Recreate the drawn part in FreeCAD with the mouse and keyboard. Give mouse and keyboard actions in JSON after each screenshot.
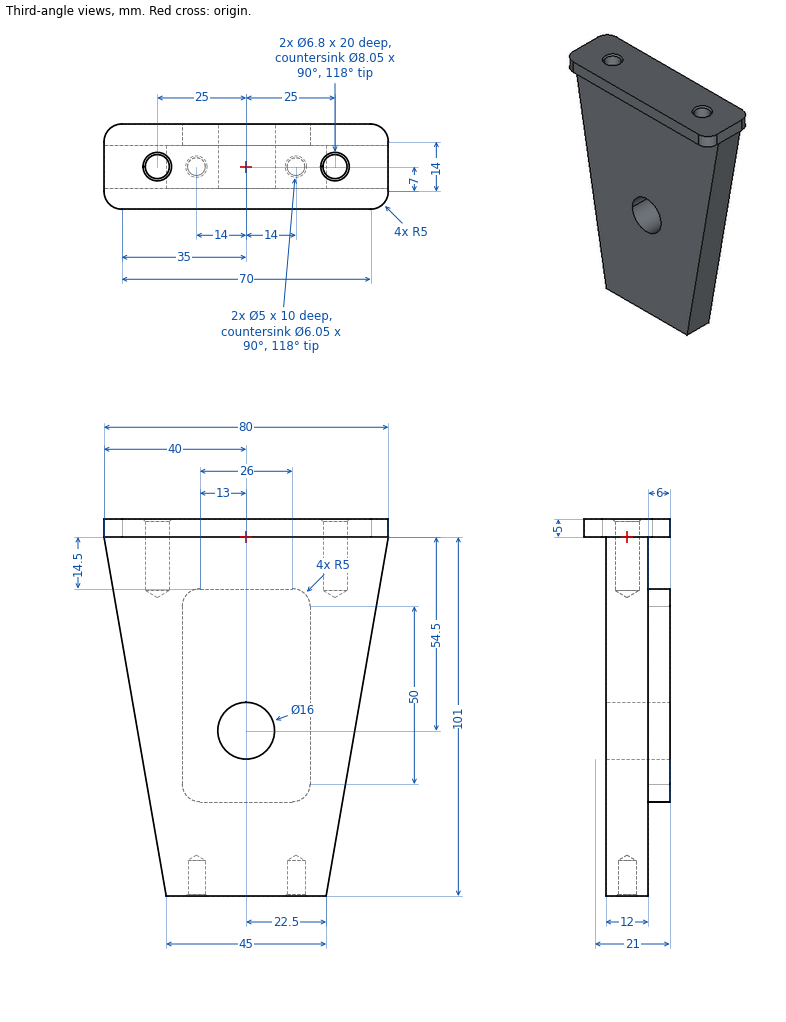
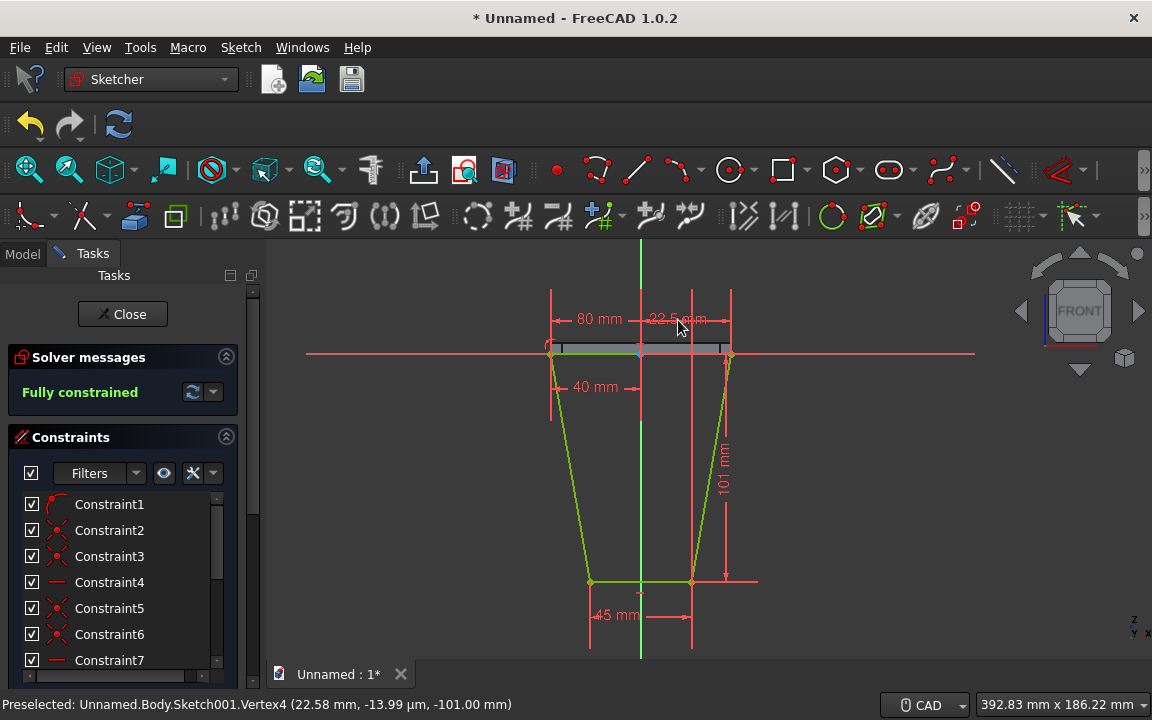
{"action": "left_click", "coordinate": [123, 314]}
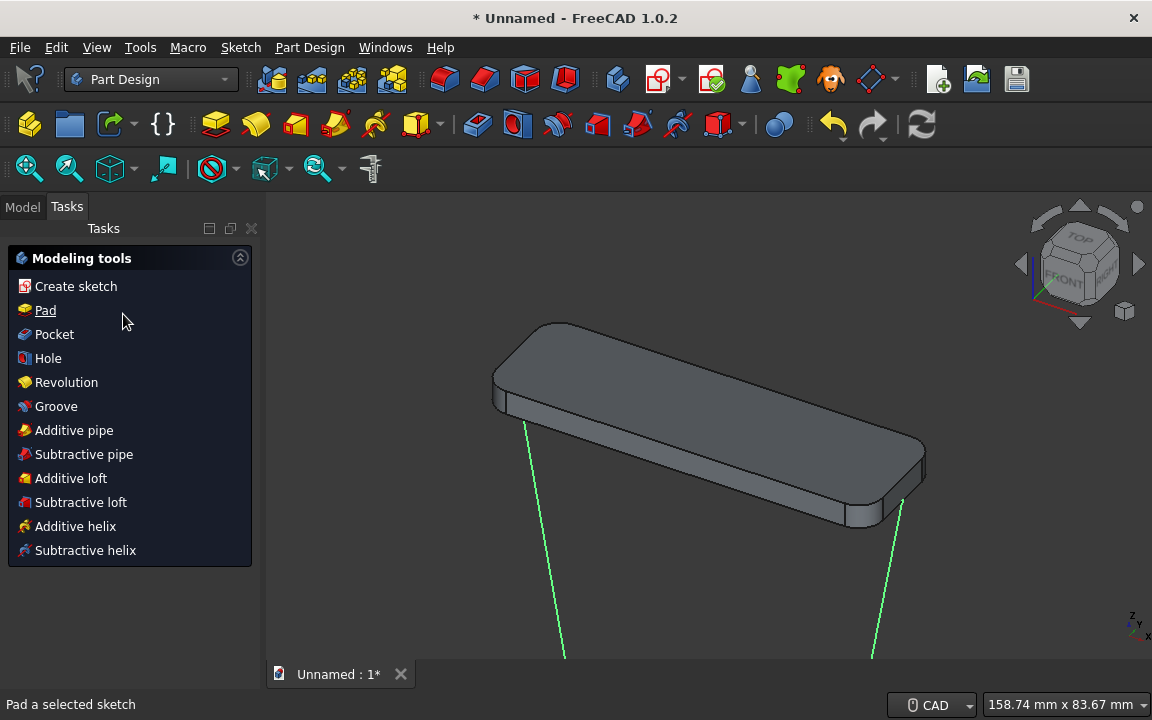
{"action": "left_click", "coordinate": [216, 124]}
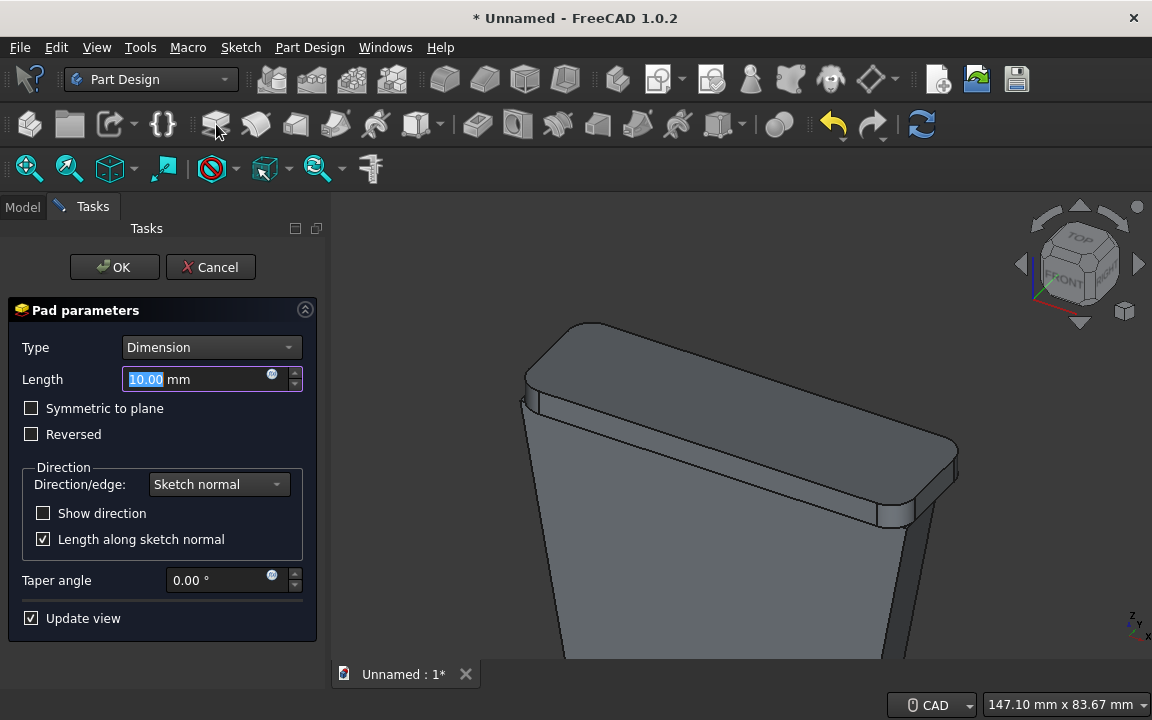
{"action": "type", "text": "12"}
{"action": "key", "text": "Tab"}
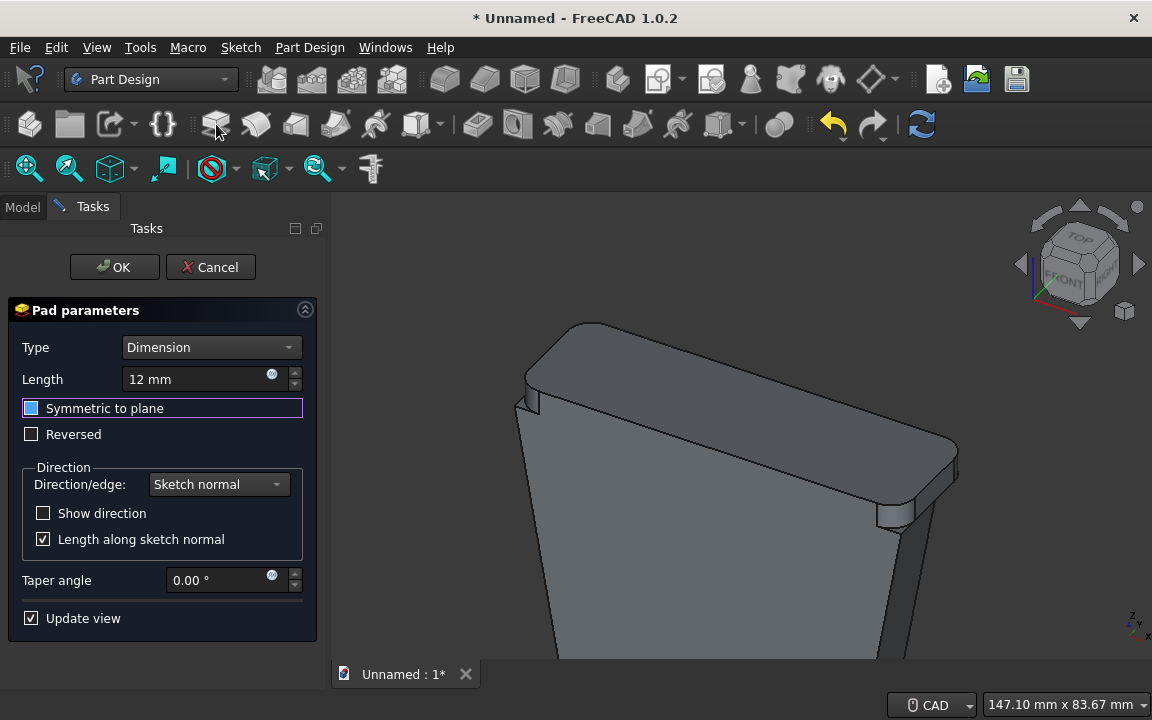
{"action": "left_click", "coordinate": [30, 408]}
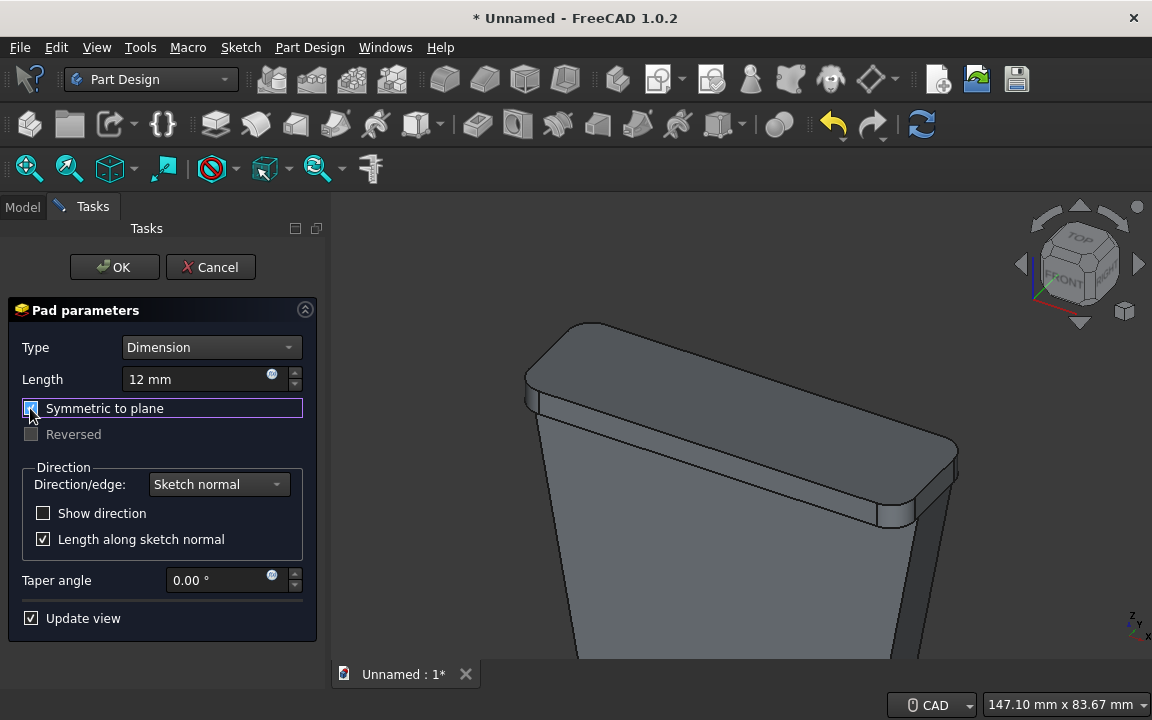
{"action": "left_click", "coordinate": [115, 267]}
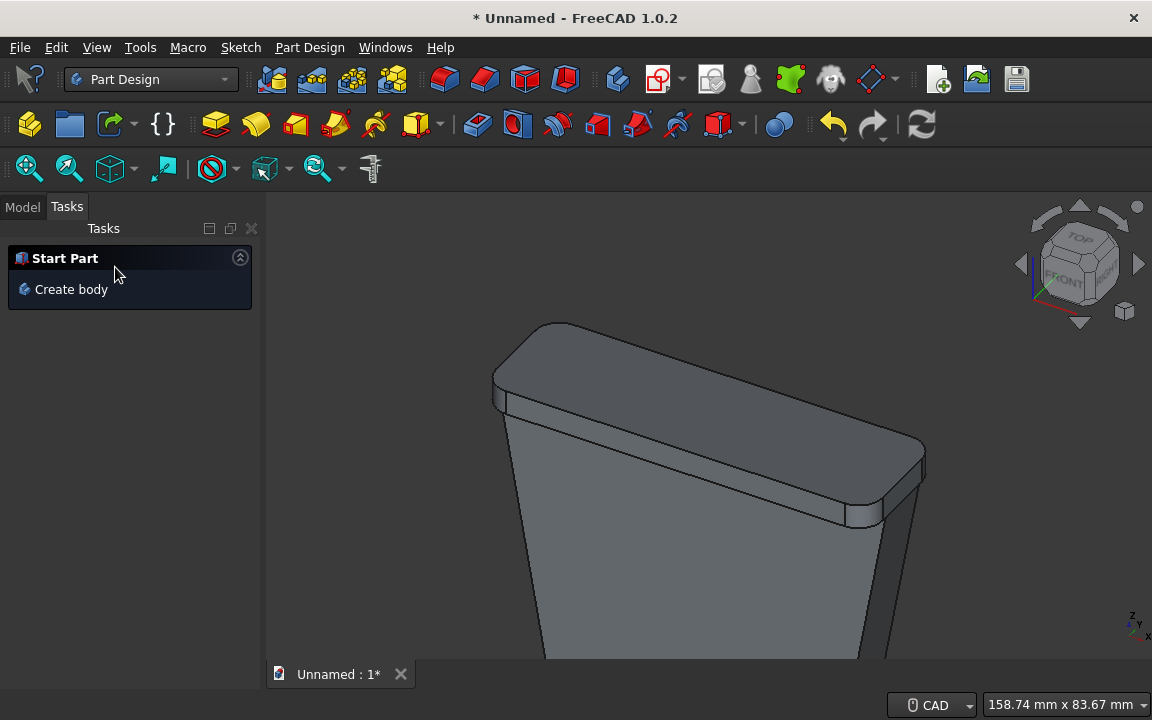
{"action": "left_click", "coordinate": [30, 170]}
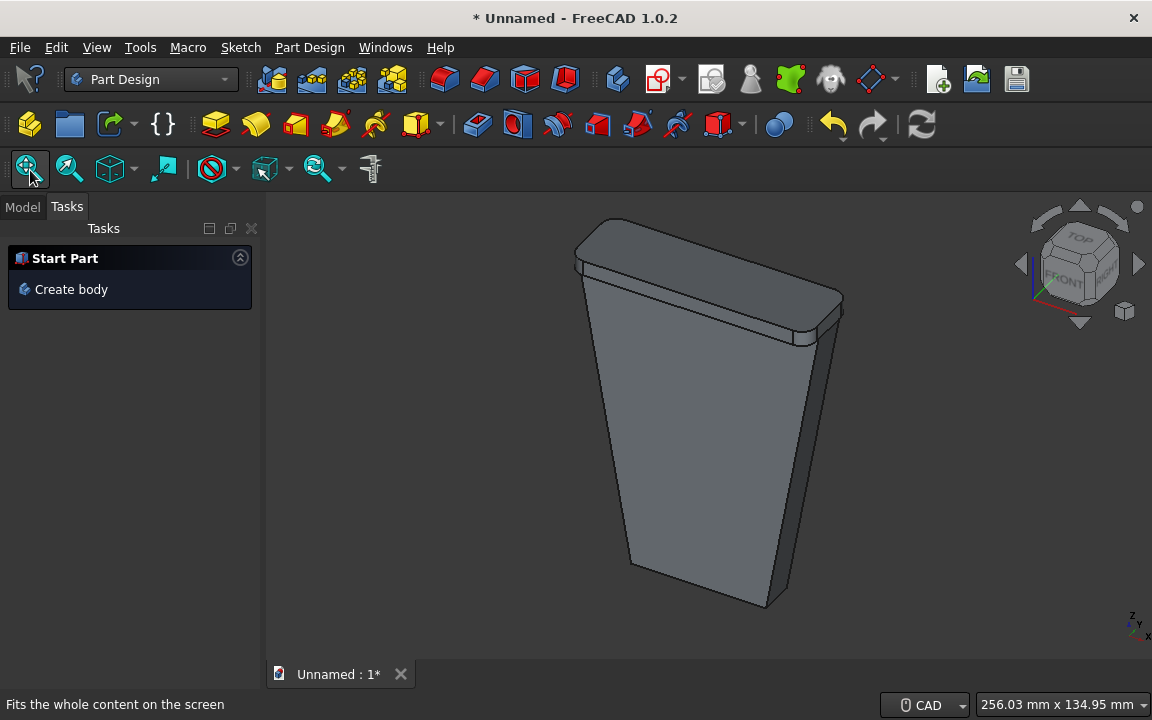
{"action": "key", "text": "4"}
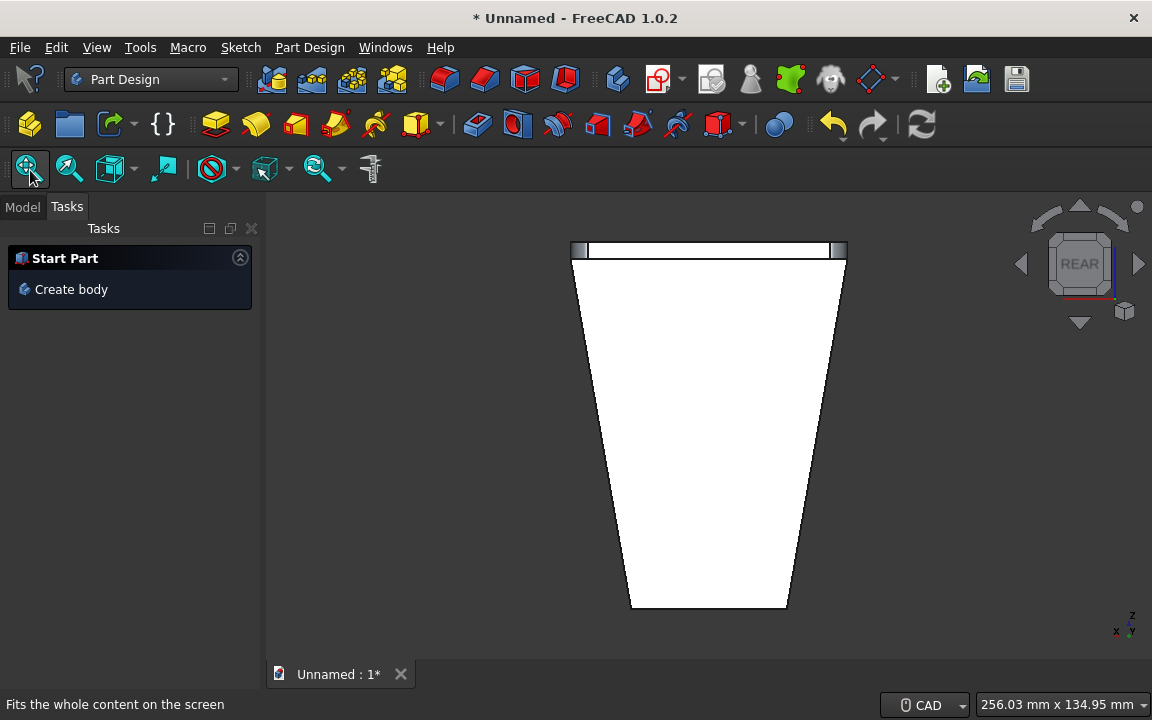
{"action": "left_click", "coordinate": [709, 383]}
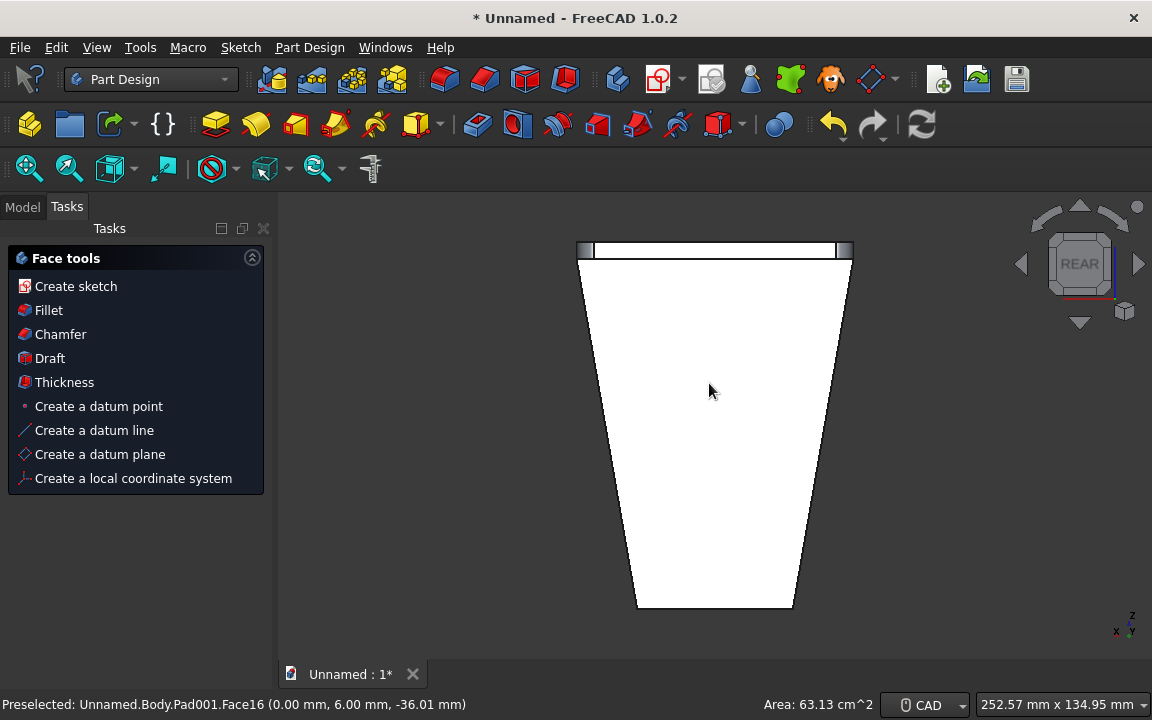
{"action": "left_click", "coordinate": [658, 80]}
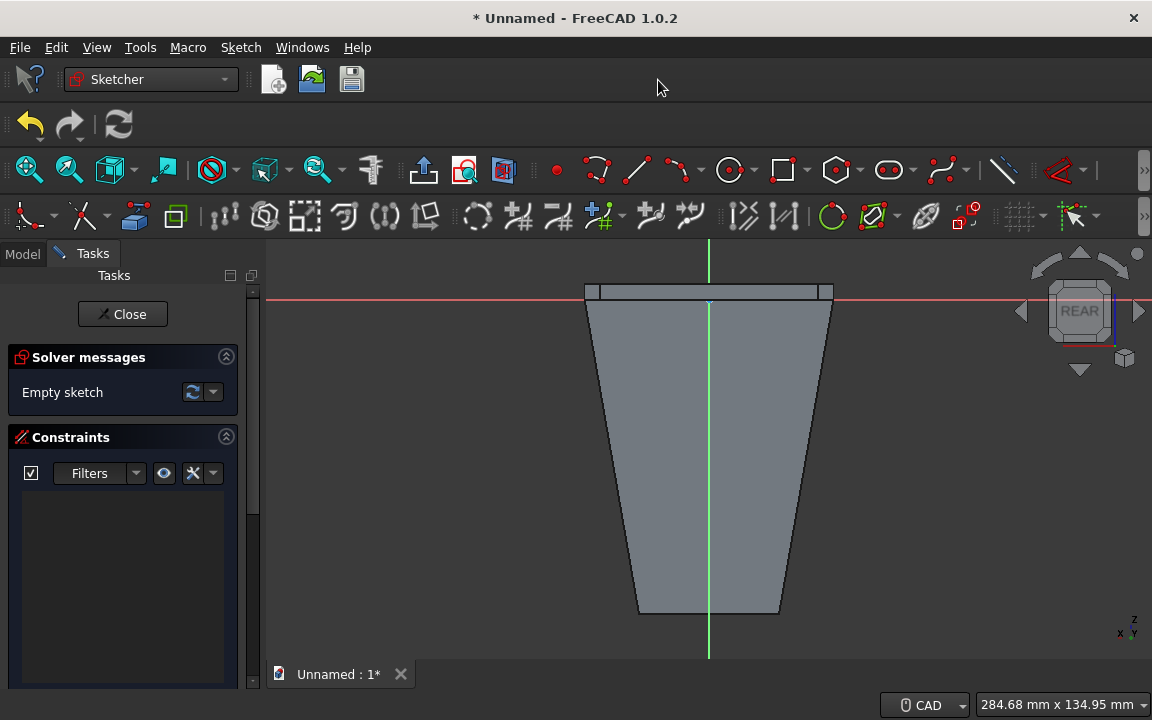
{"action": "left_click", "coordinate": [504, 170]}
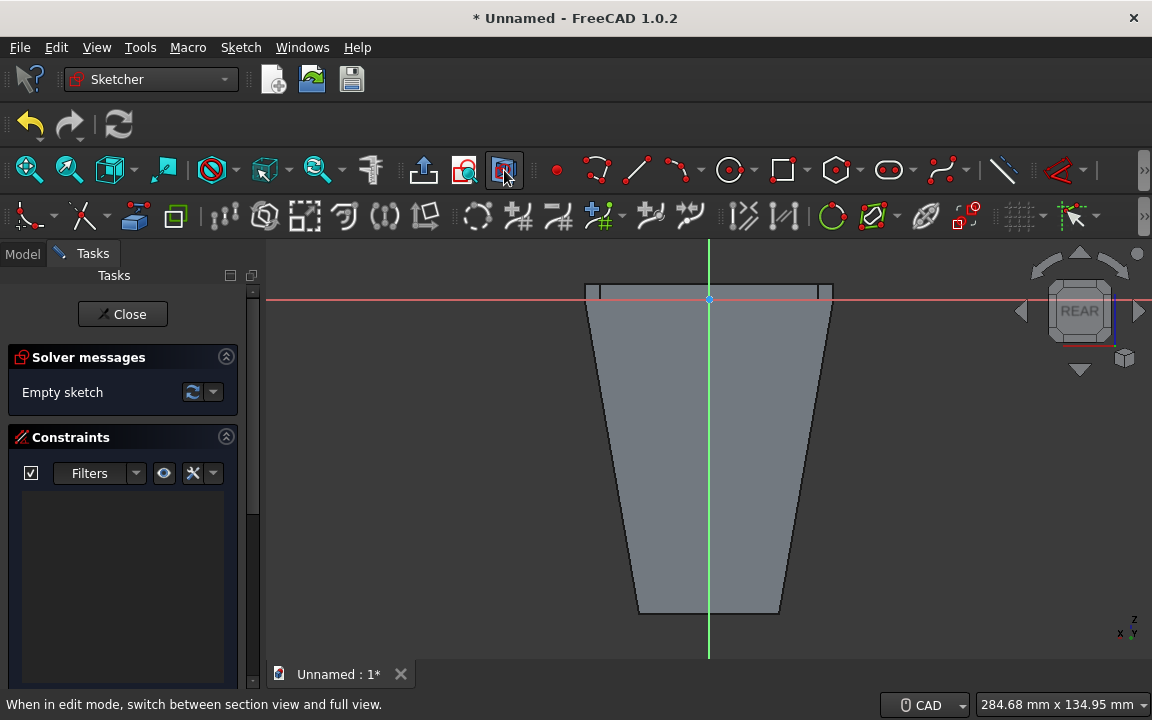
{"action": "left_click", "coordinate": [638, 170]}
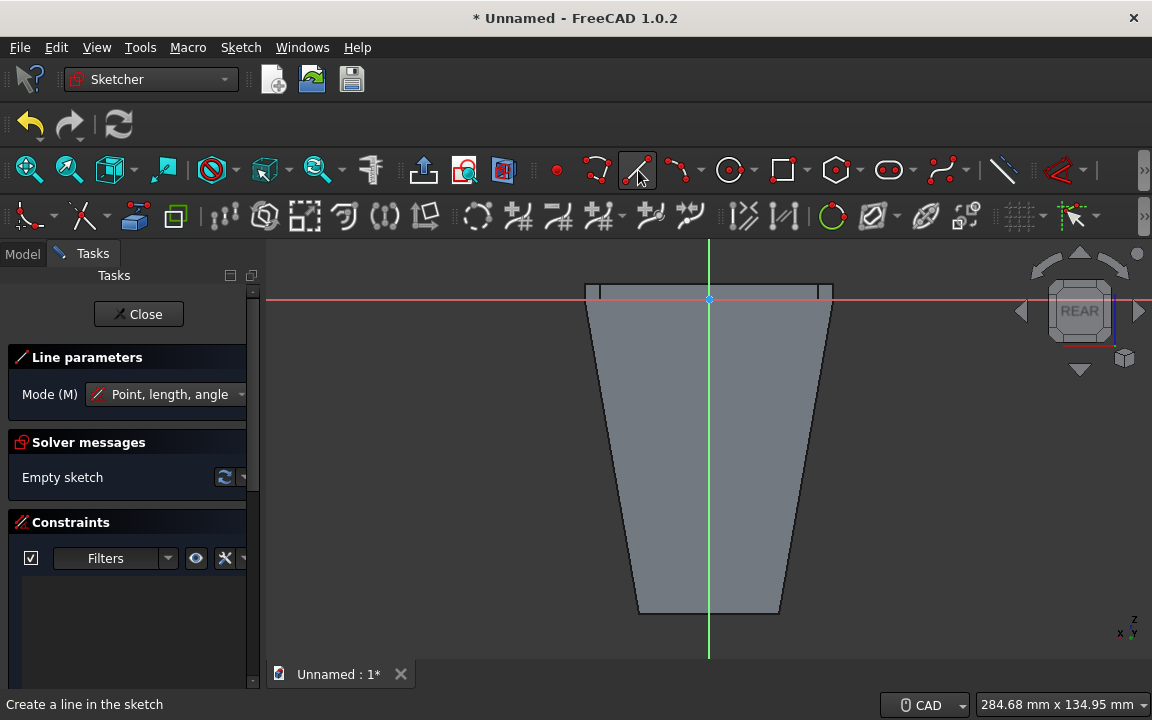
{"action": "left_click", "coordinate": [749, 345]}
{"action": "left_click", "coordinate": [669, 345]}